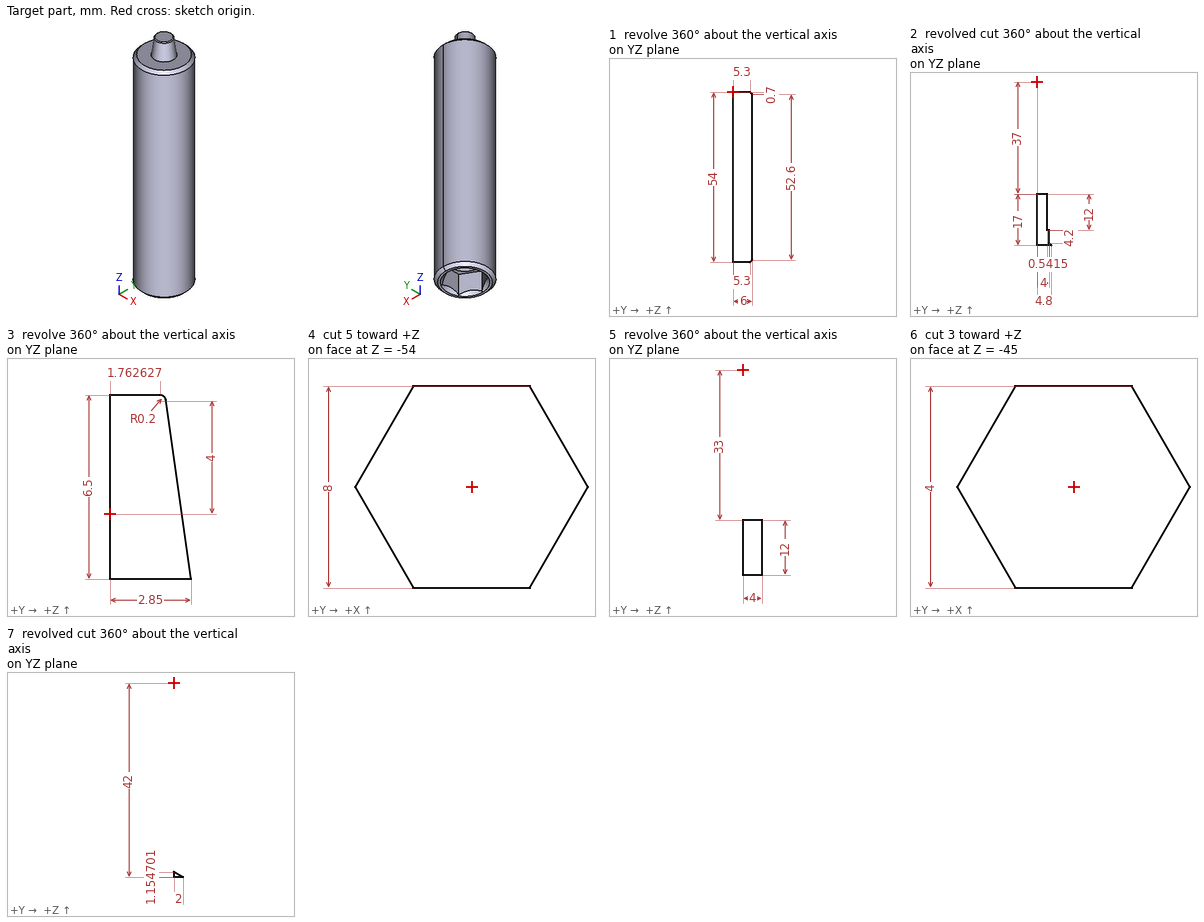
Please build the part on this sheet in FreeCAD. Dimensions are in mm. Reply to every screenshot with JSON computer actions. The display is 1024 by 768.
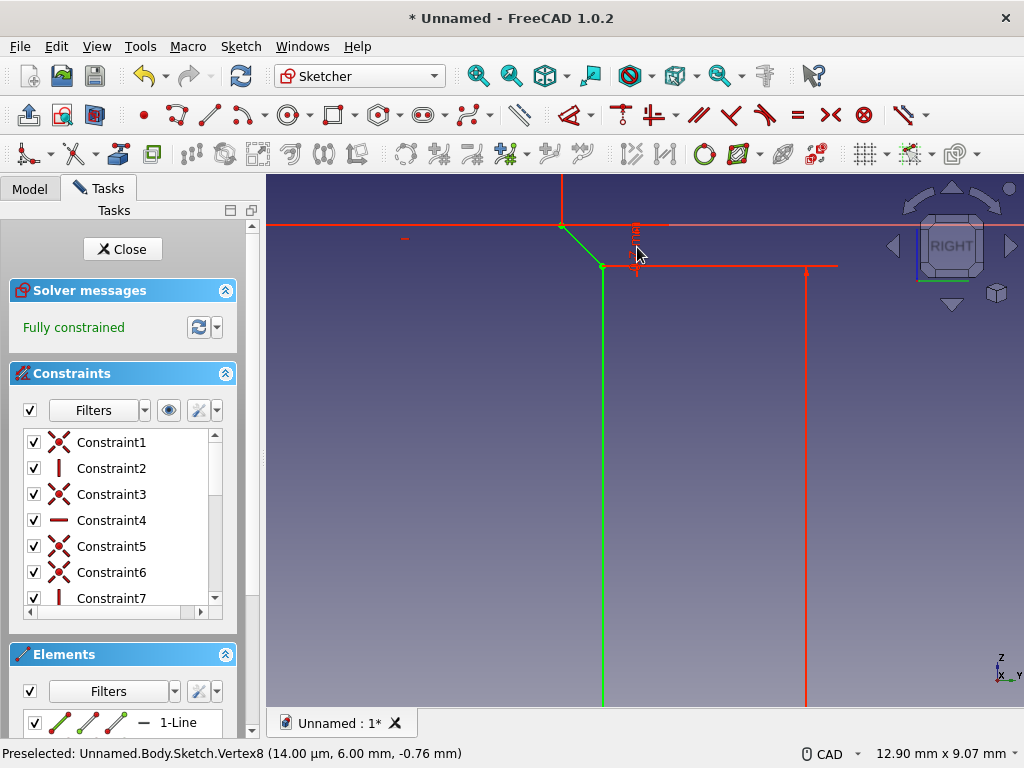
{"action": "left_click", "coordinate": [123, 249]}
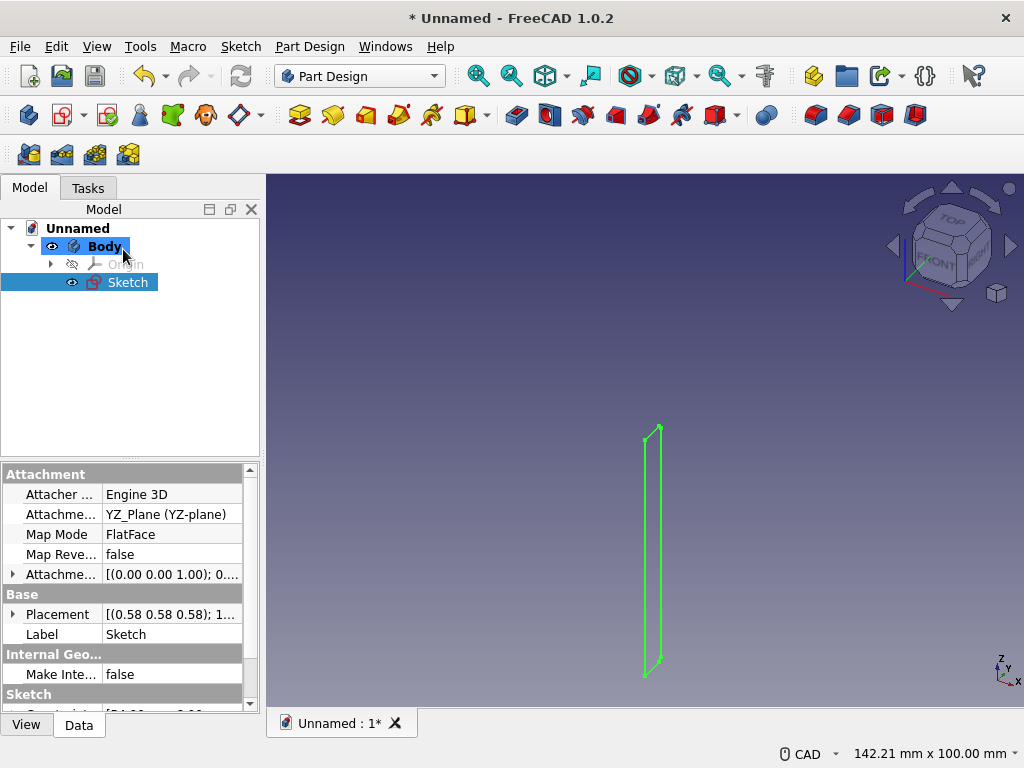
{"action": "left_click", "coordinate": [333, 116]}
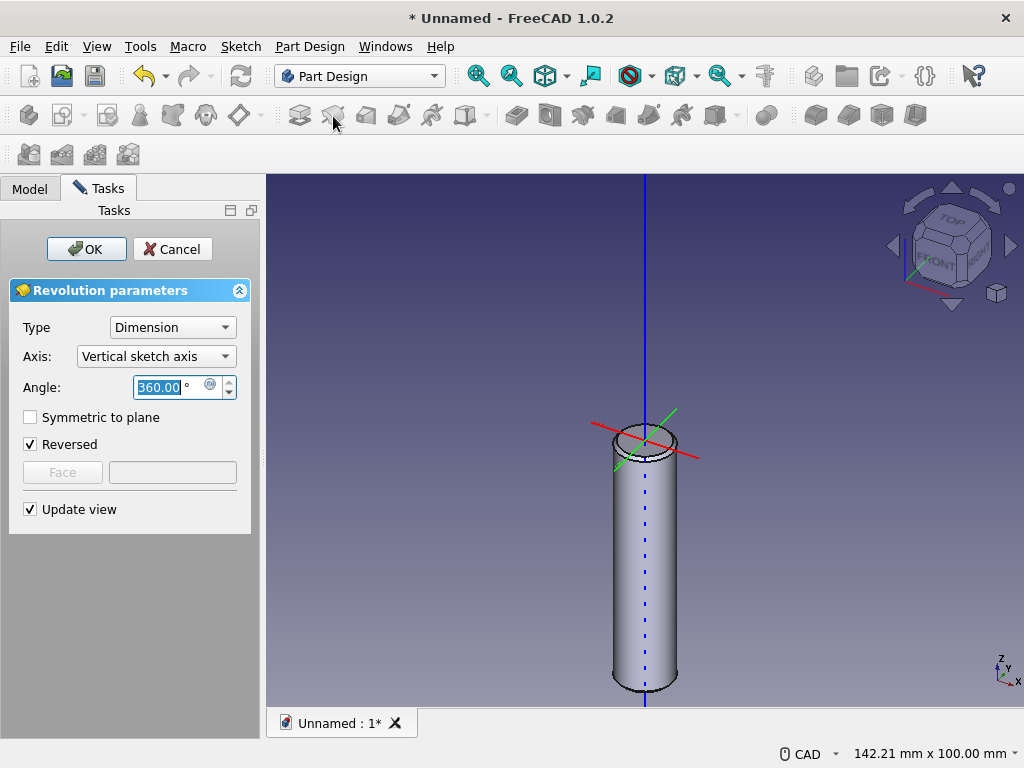
{"action": "left_click", "coordinate": [87, 249]}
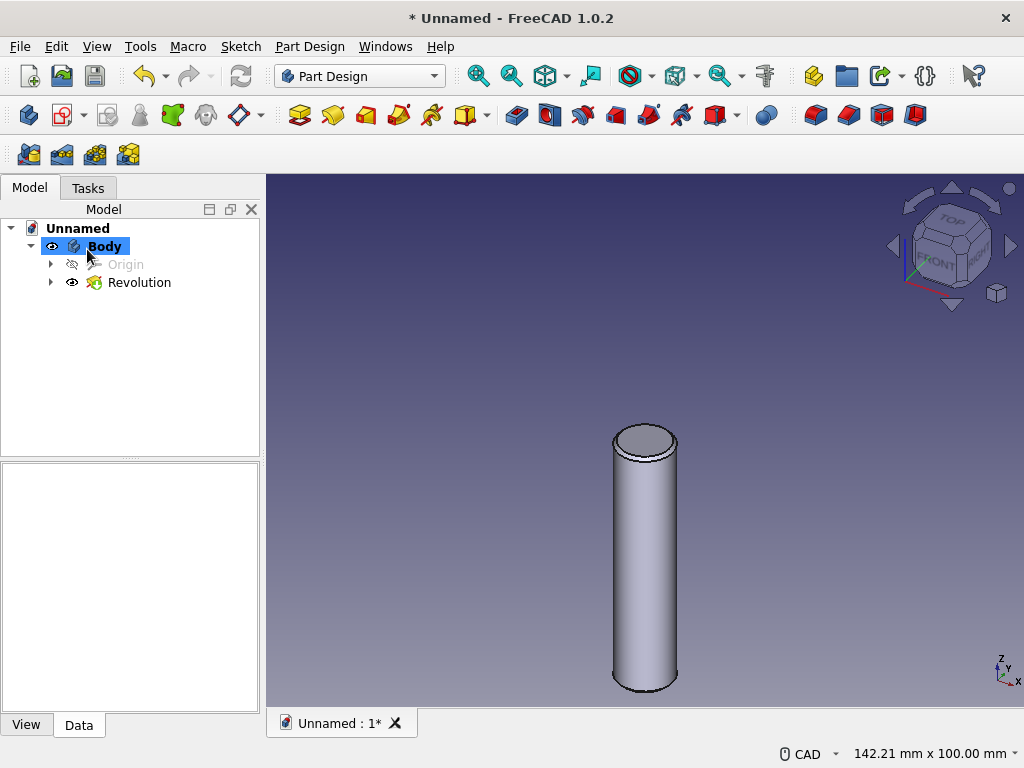
{"action": "left_click", "coordinate": [62, 116]}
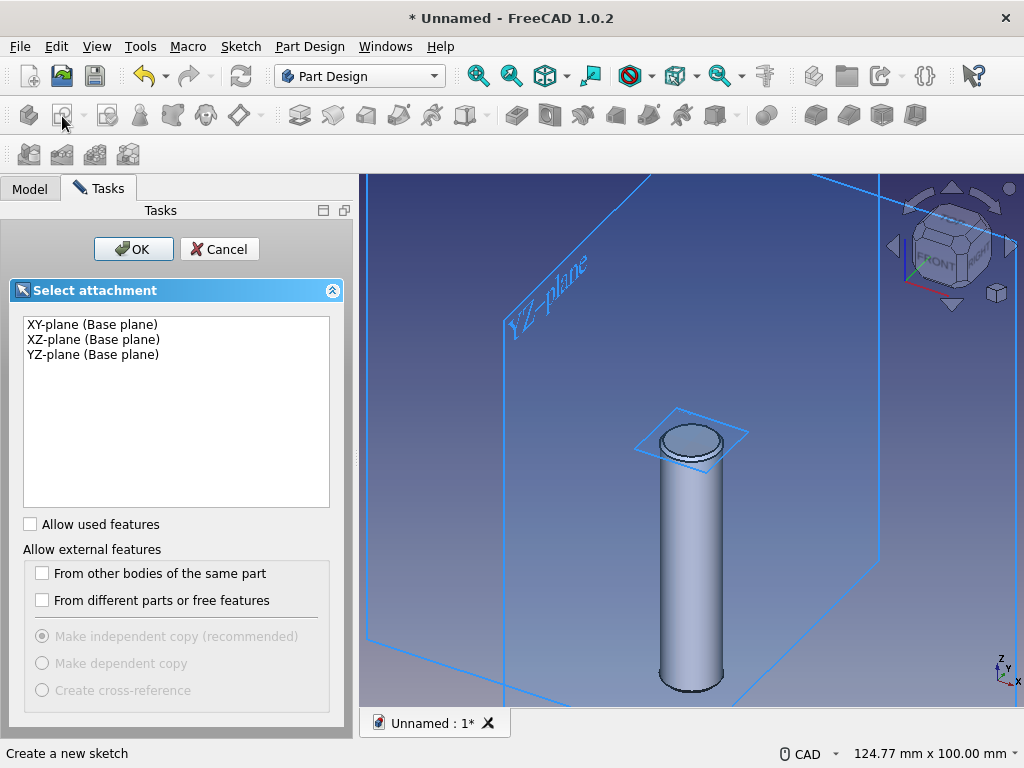
{"action": "left_click", "coordinate": [84, 354]}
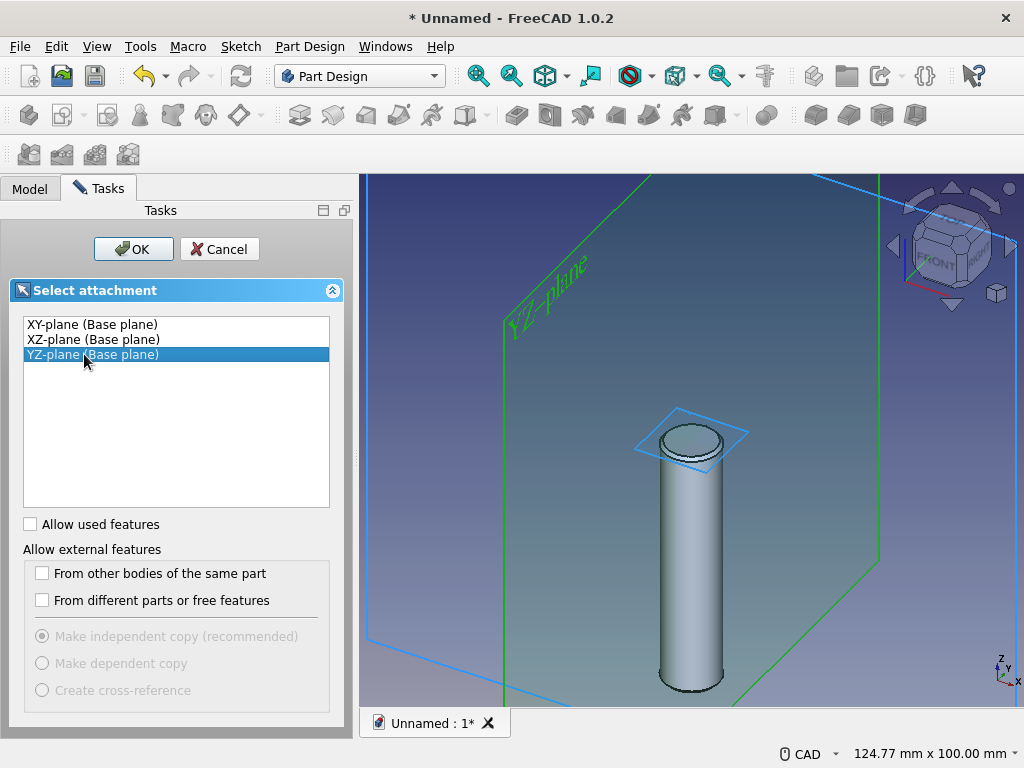
{"action": "left_click", "coordinate": [134, 249]}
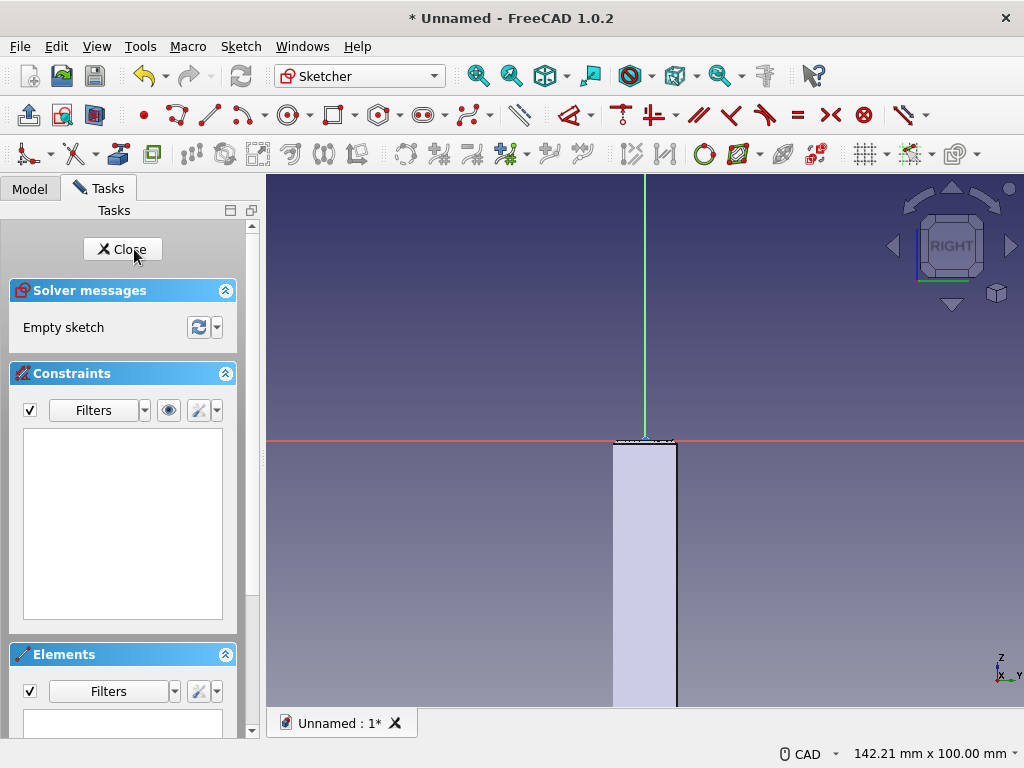
{"action": "left_click", "coordinate": [95, 116]}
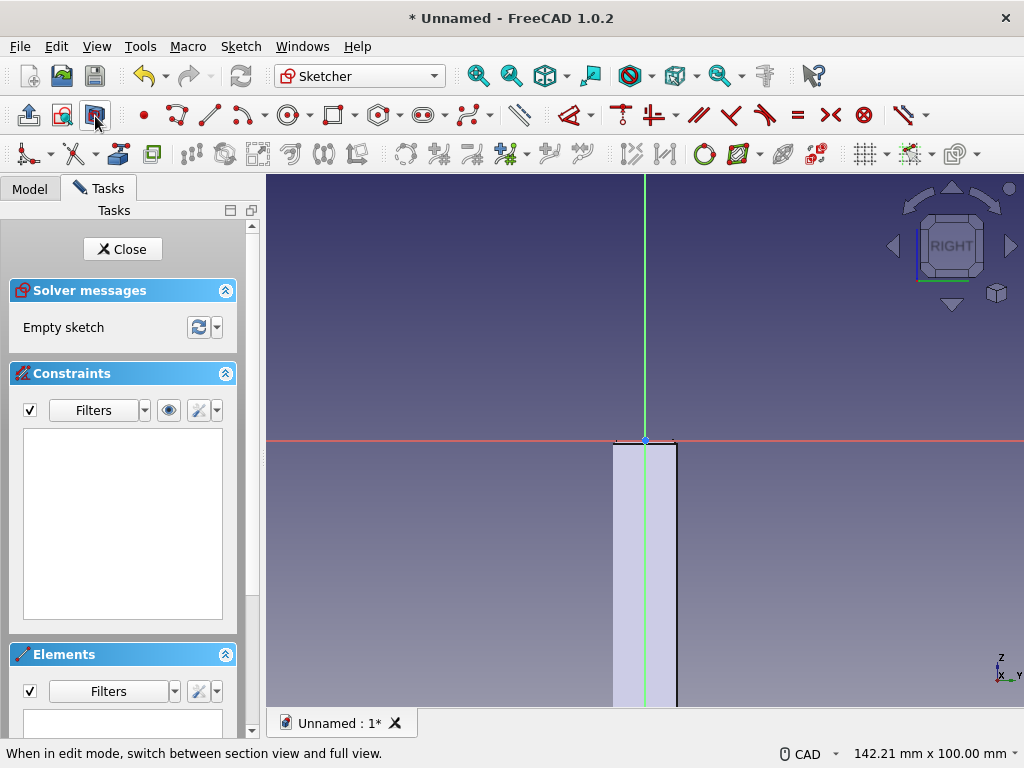
{"action": "scroll", "coordinate": [576, 440], "scroll_direction": "down", "scroll_amount": 5}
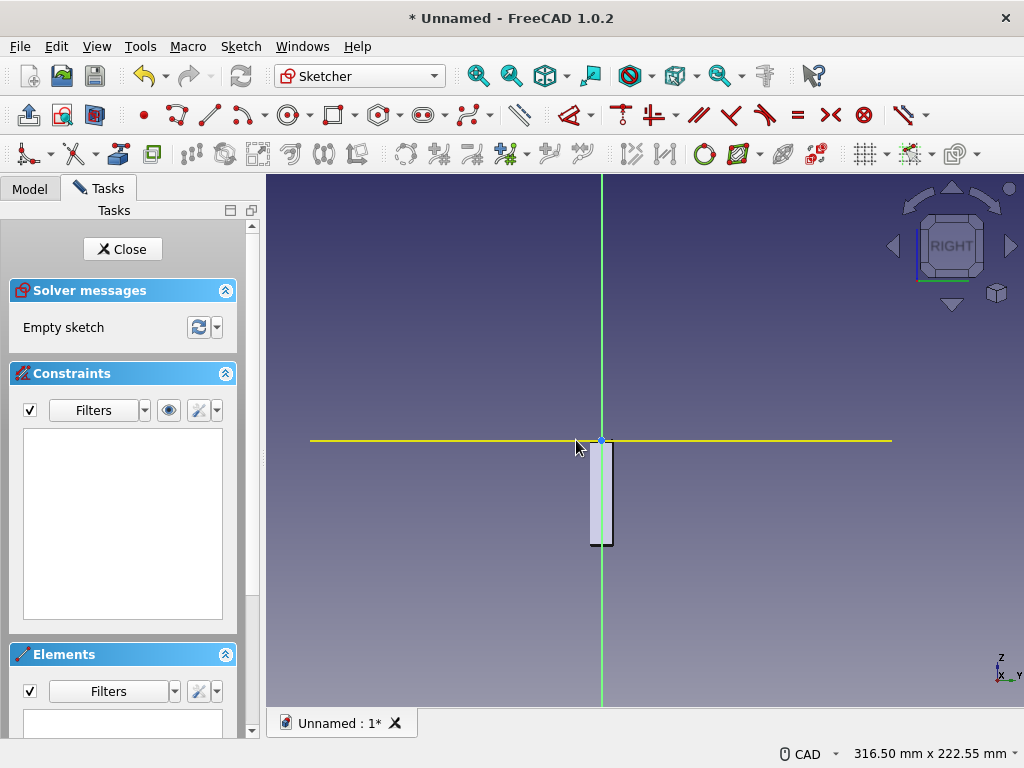
{"action": "scroll", "coordinate": [609, 539], "scroll_direction": "up", "scroll_amount": 12}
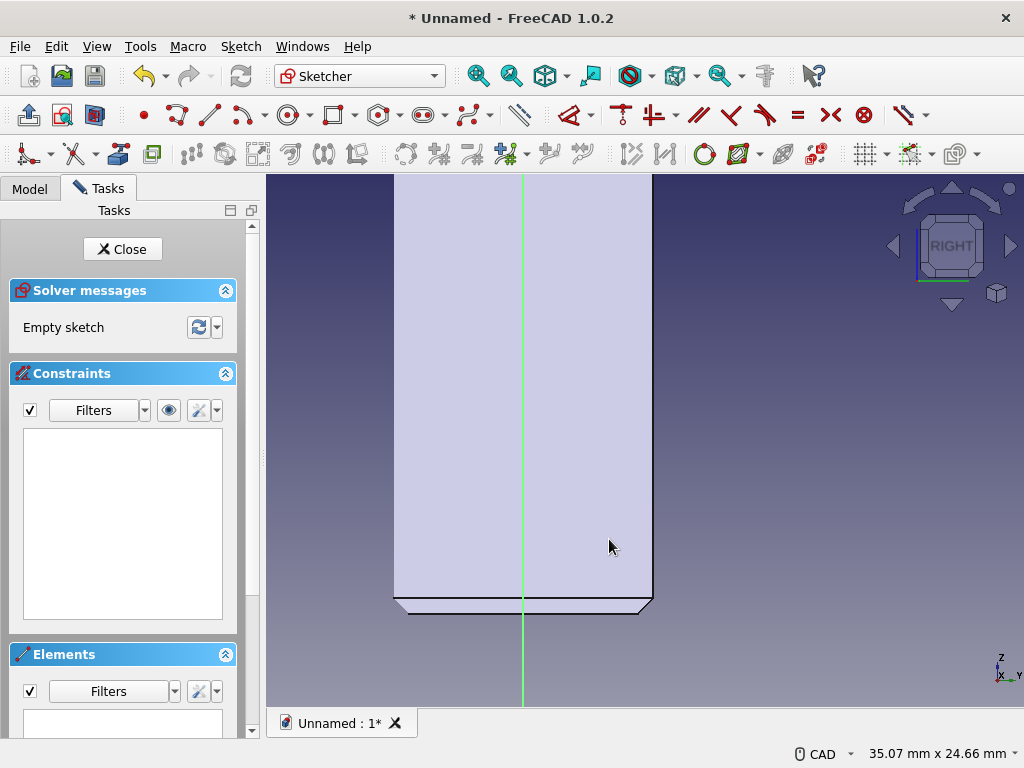
{"action": "left_click", "coordinate": [177, 116]}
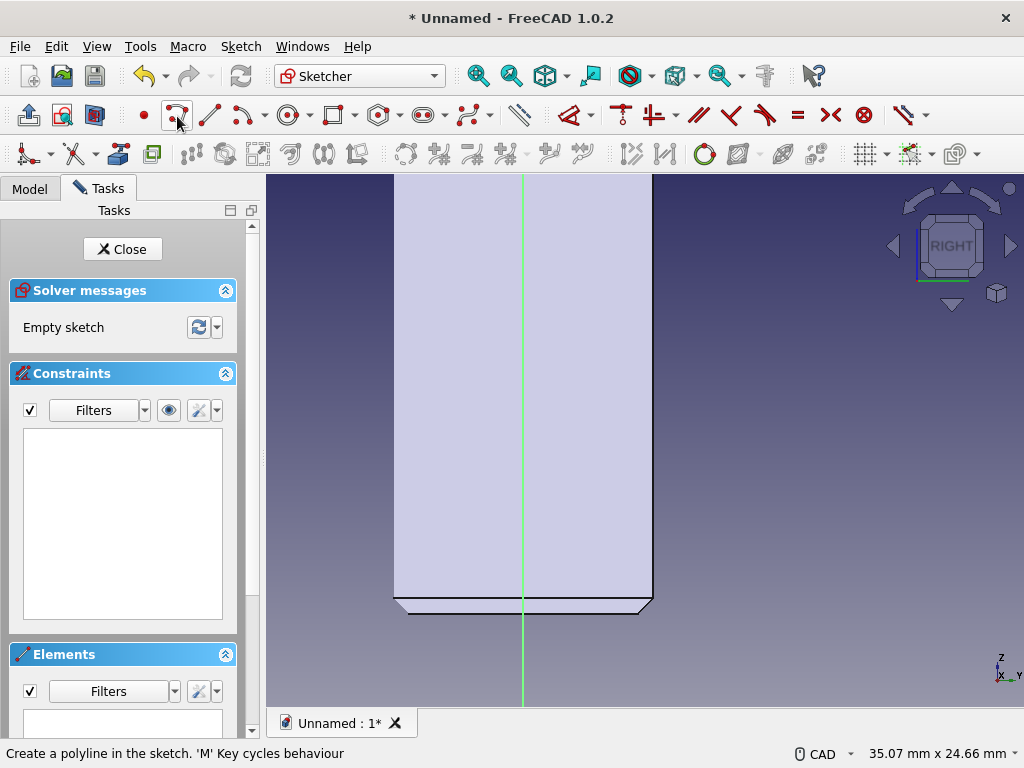
{"action": "left_click", "coordinate": [523, 246]}
{"action": "left_click", "coordinate": [532, 614]}
{"action": "left_click", "coordinate": [627, 614]}
{"action": "left_click", "coordinate": [610, 596]}
{"action": "left_click", "coordinate": [610, 505]}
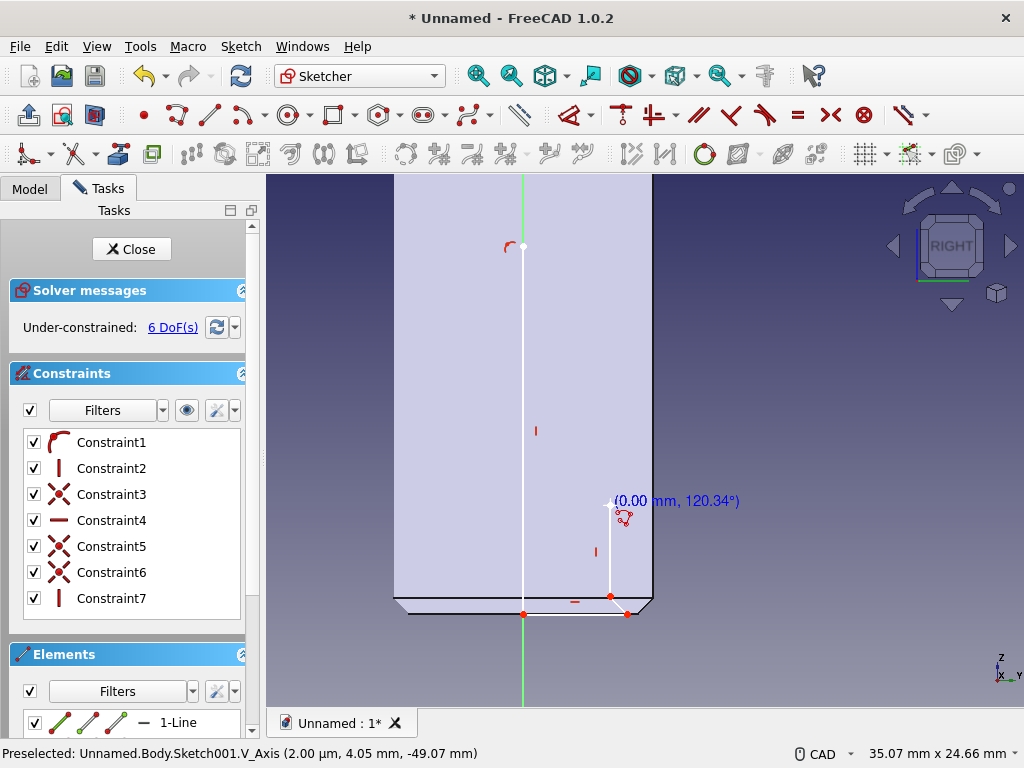
{"action": "scroll", "coordinate": [598, 505], "scroll_direction": "up", "scroll_amount": 2}